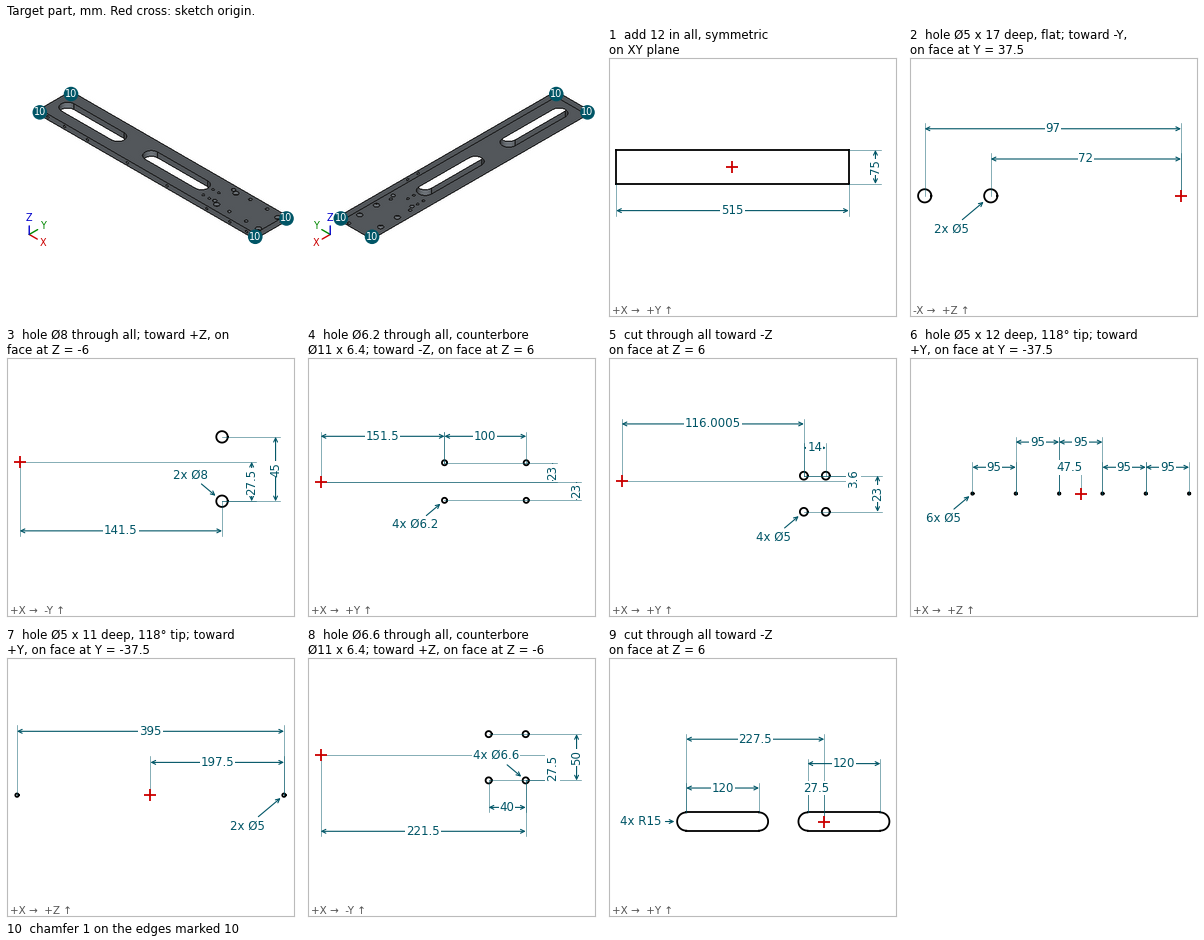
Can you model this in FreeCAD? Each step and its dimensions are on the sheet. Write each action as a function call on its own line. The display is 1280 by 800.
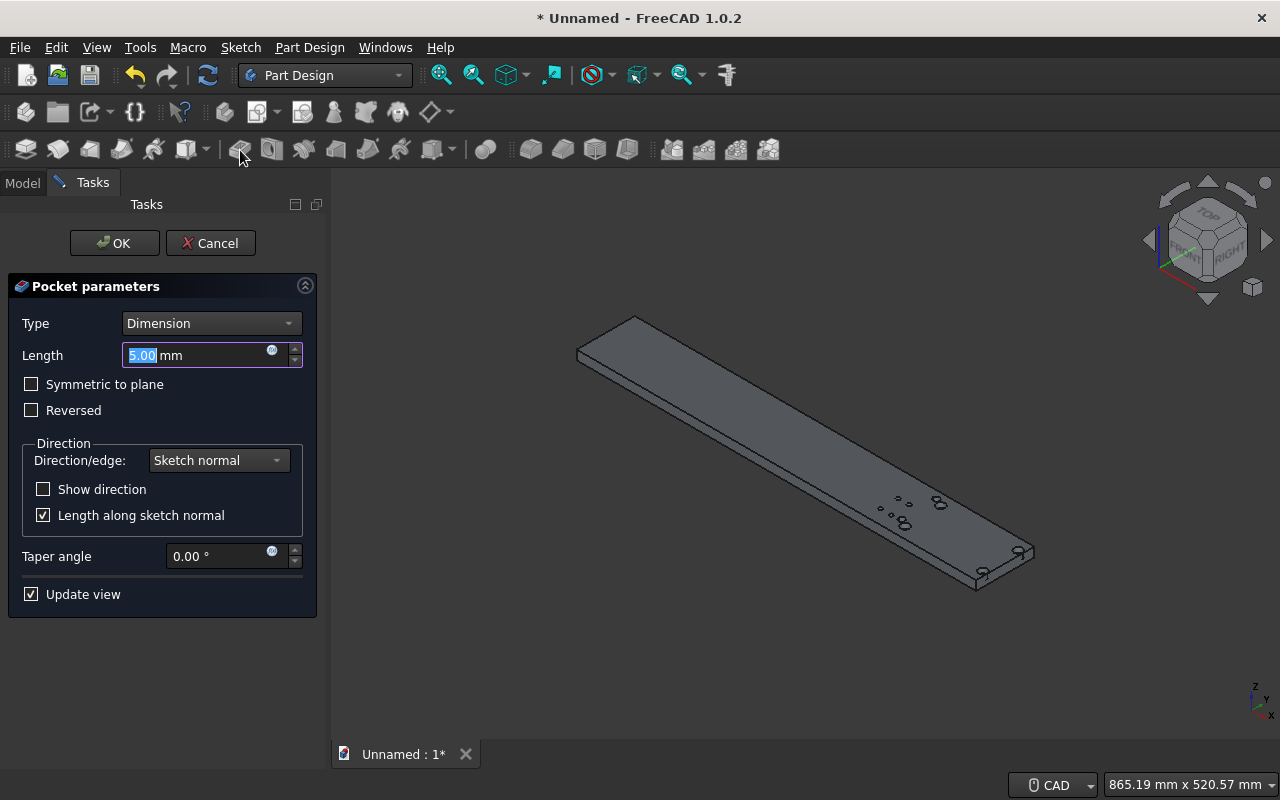
click(212, 324)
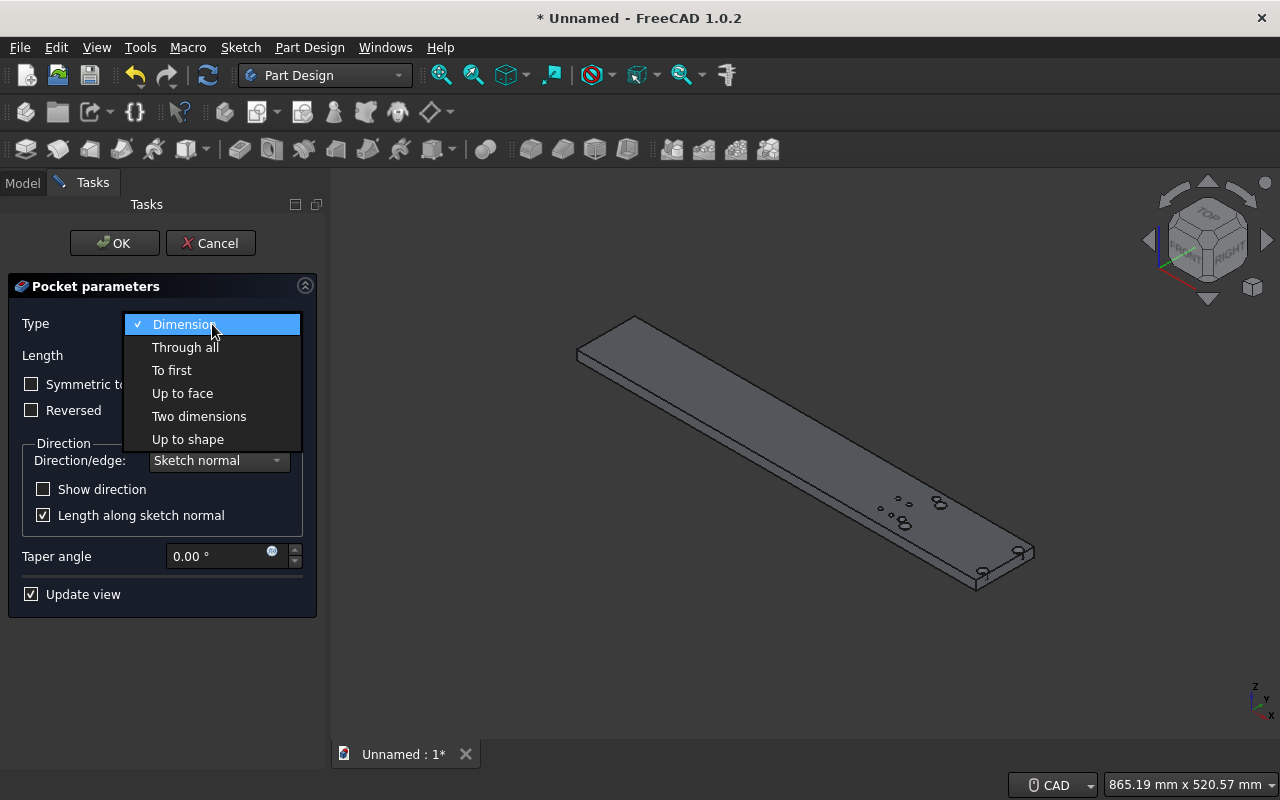
click(212, 348)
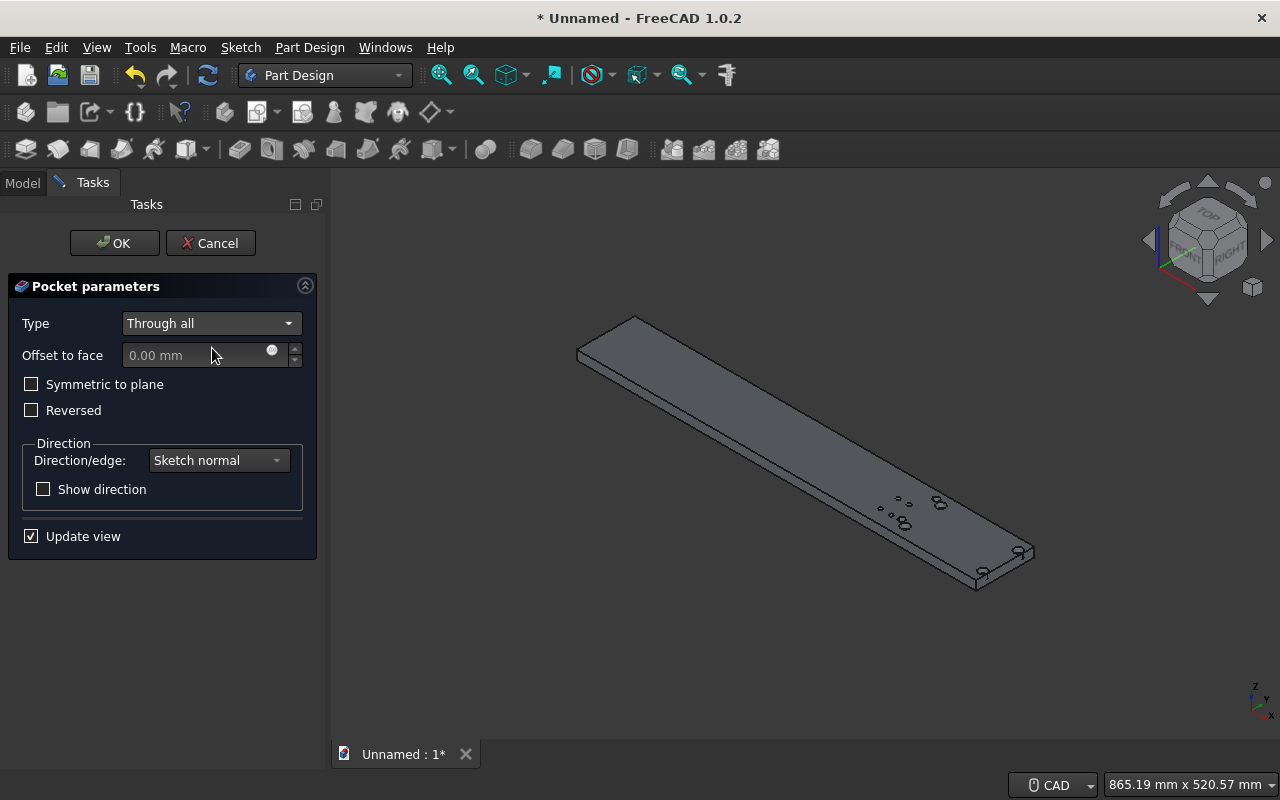
click(115, 243)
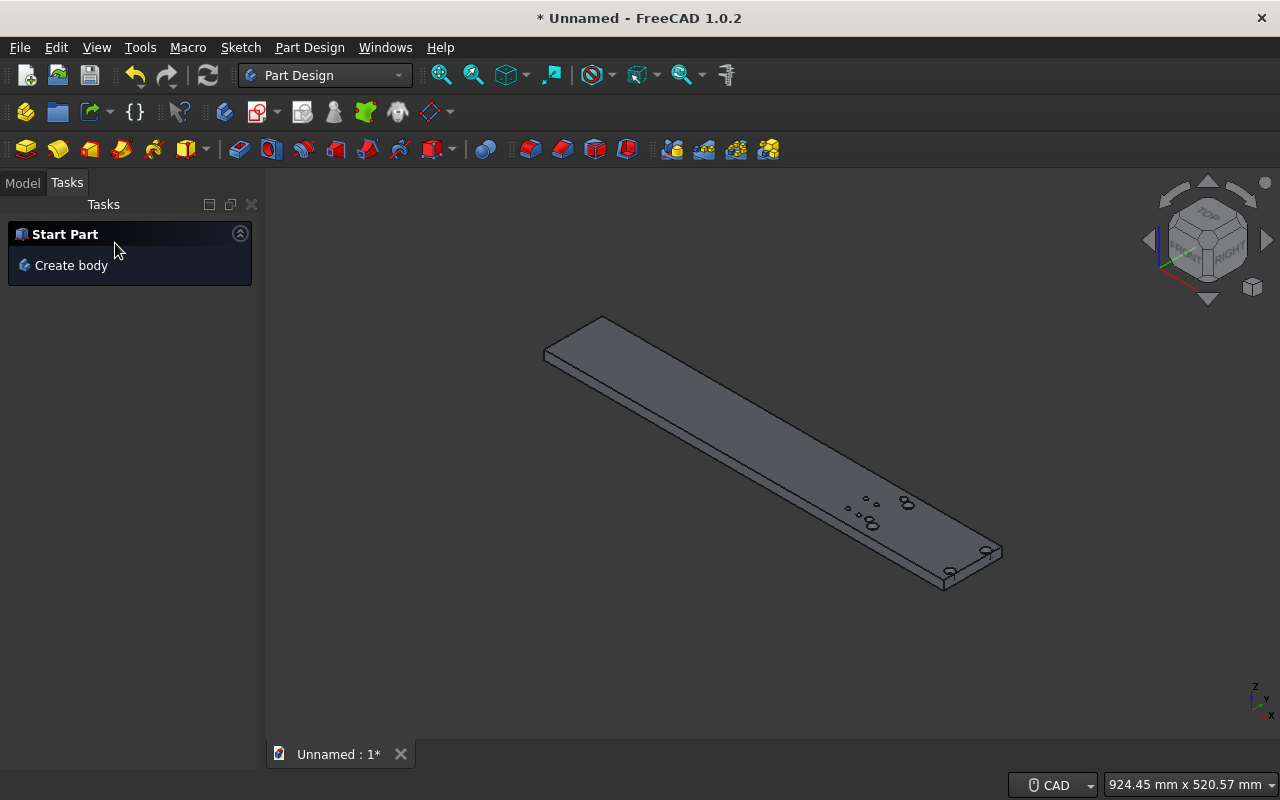
scroll(915, 568, up, 4)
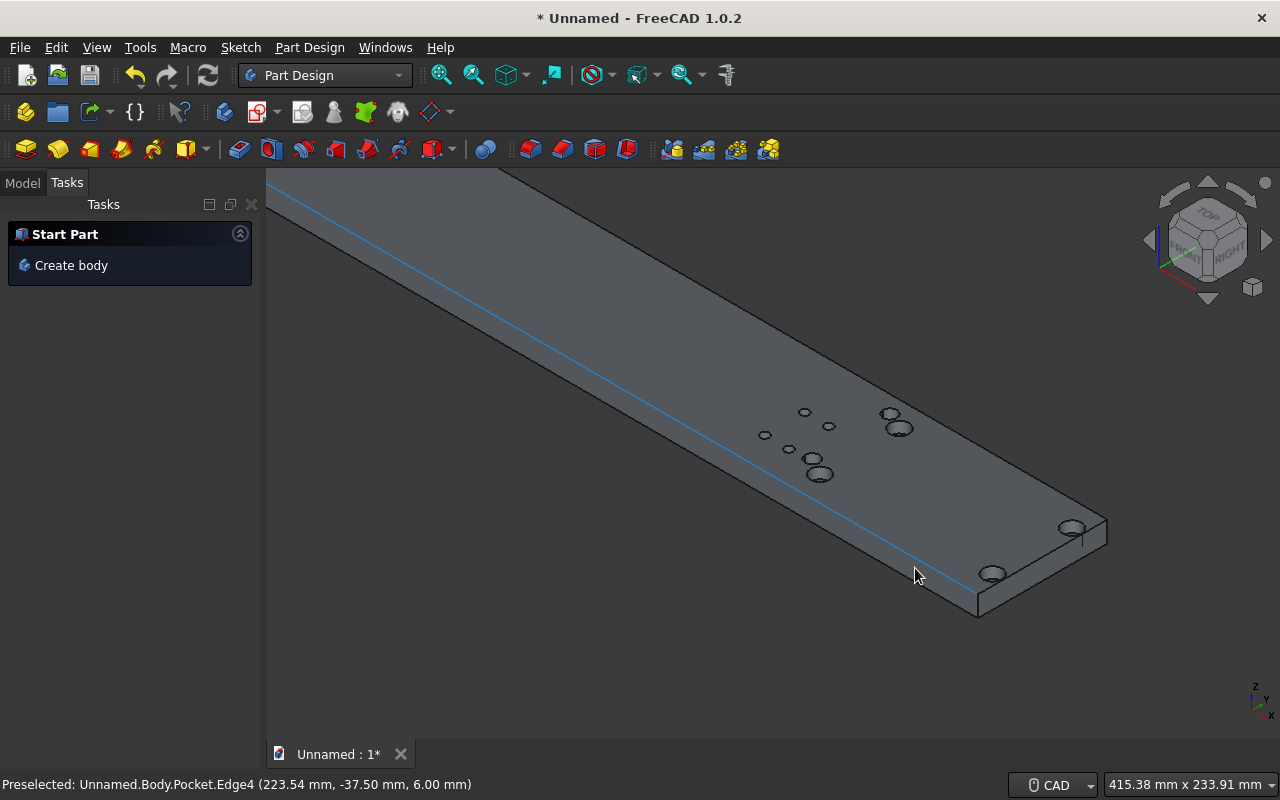
click(914, 569)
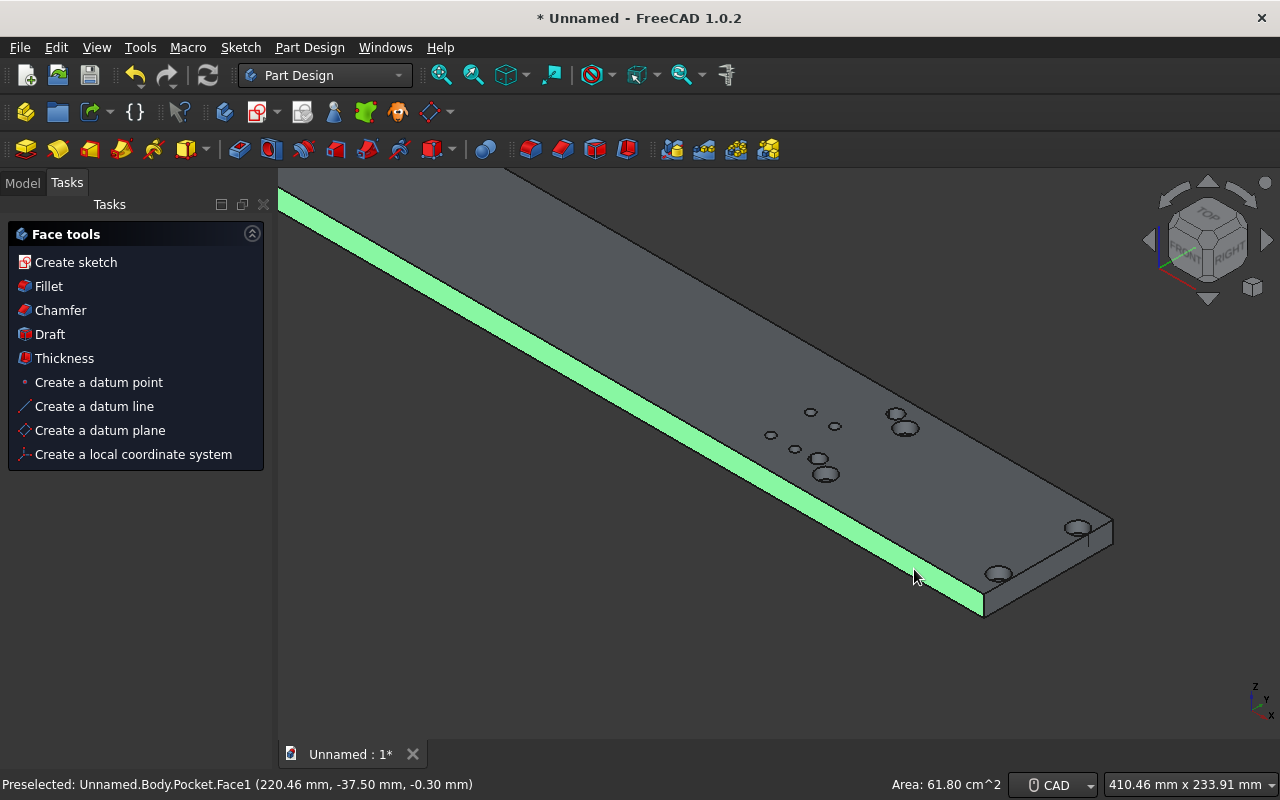
click(258, 112)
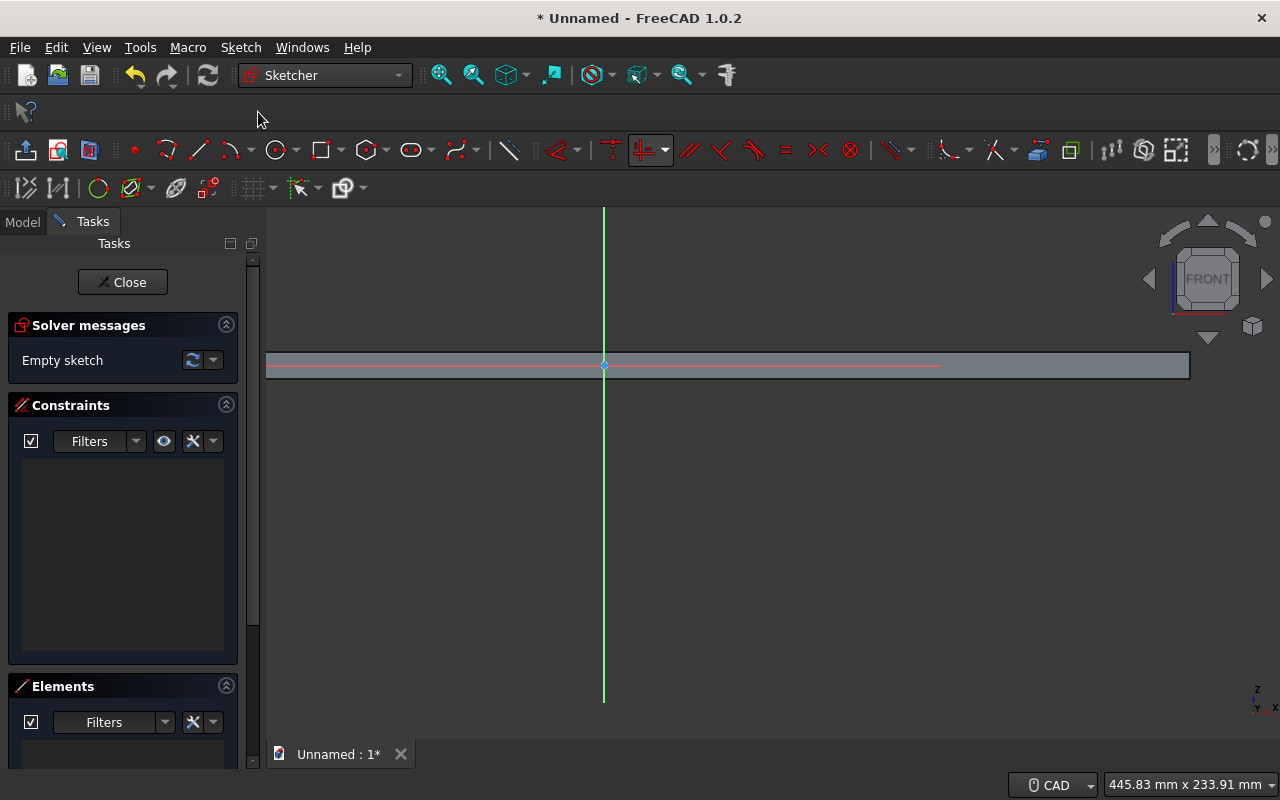
scroll(827, 604, down, 3)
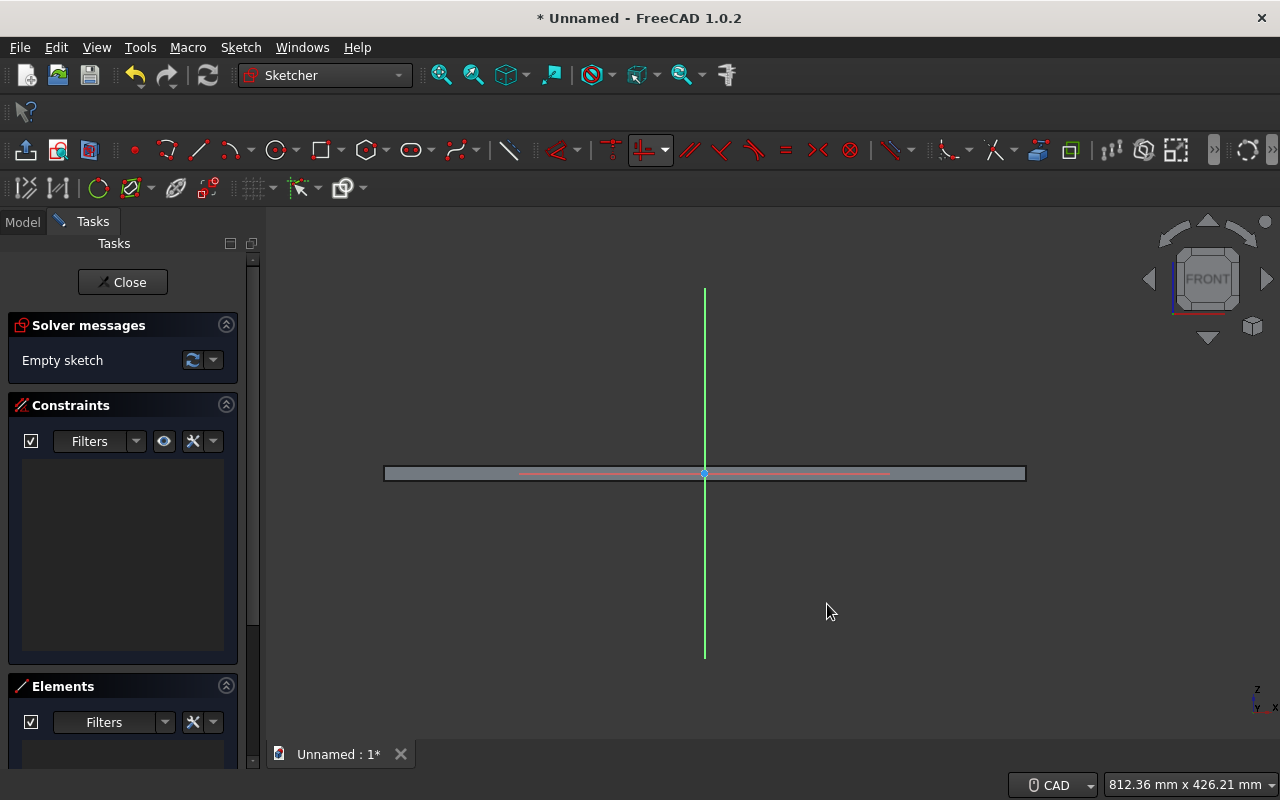
click(276, 150)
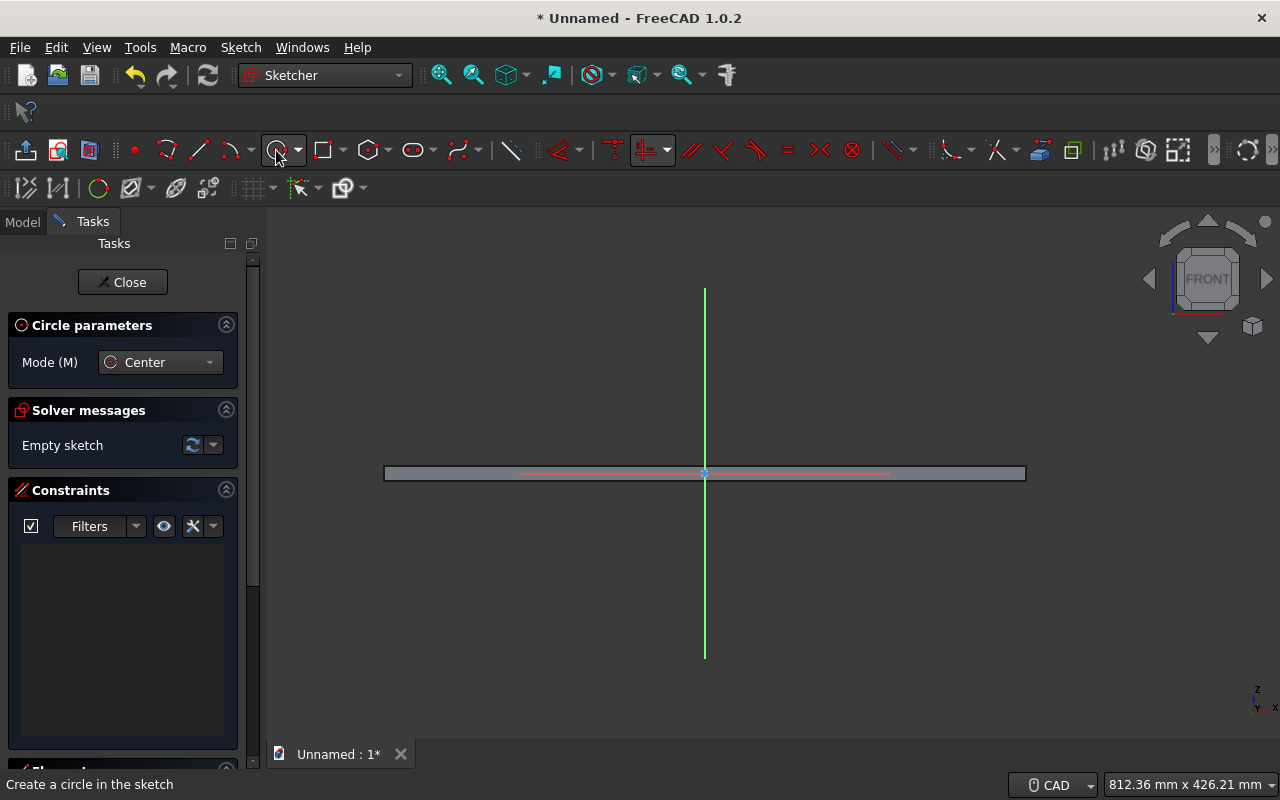
scroll(408, 473, up, 10)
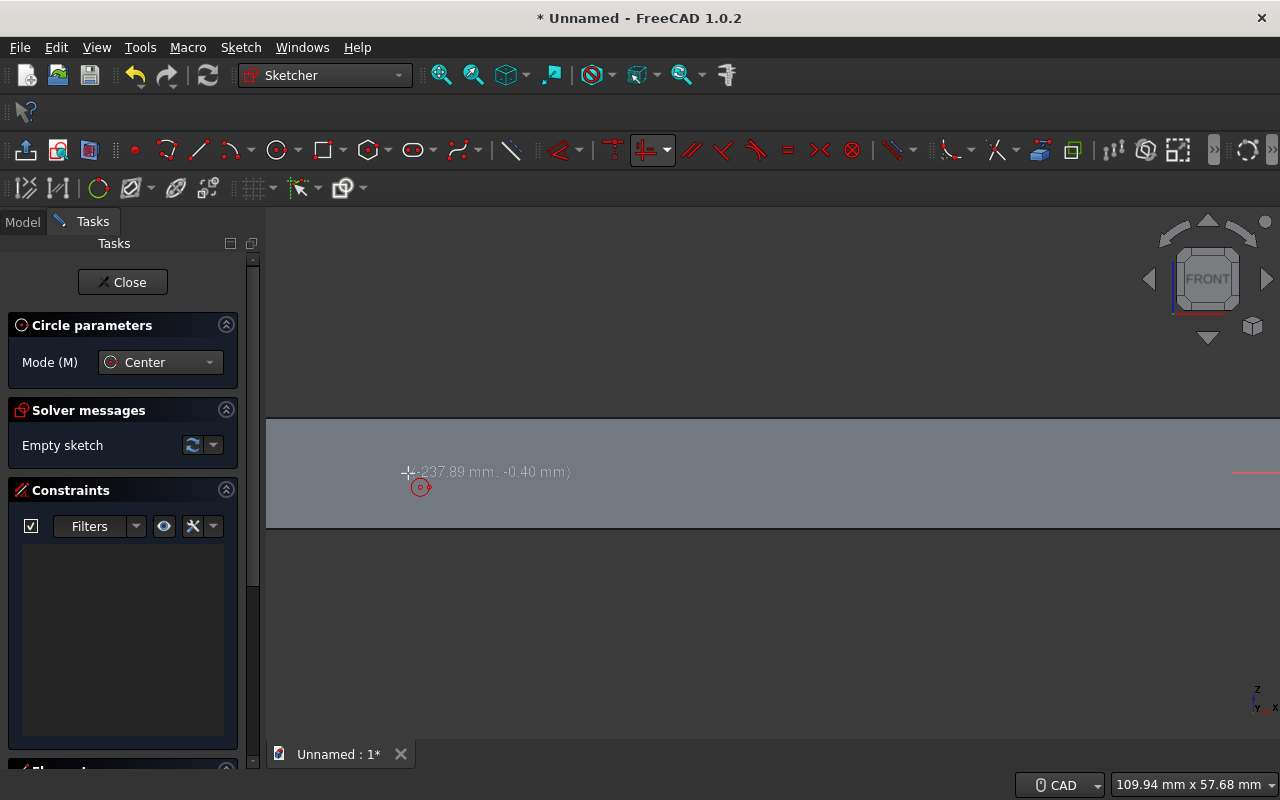
scroll(408, 473, down, 10)